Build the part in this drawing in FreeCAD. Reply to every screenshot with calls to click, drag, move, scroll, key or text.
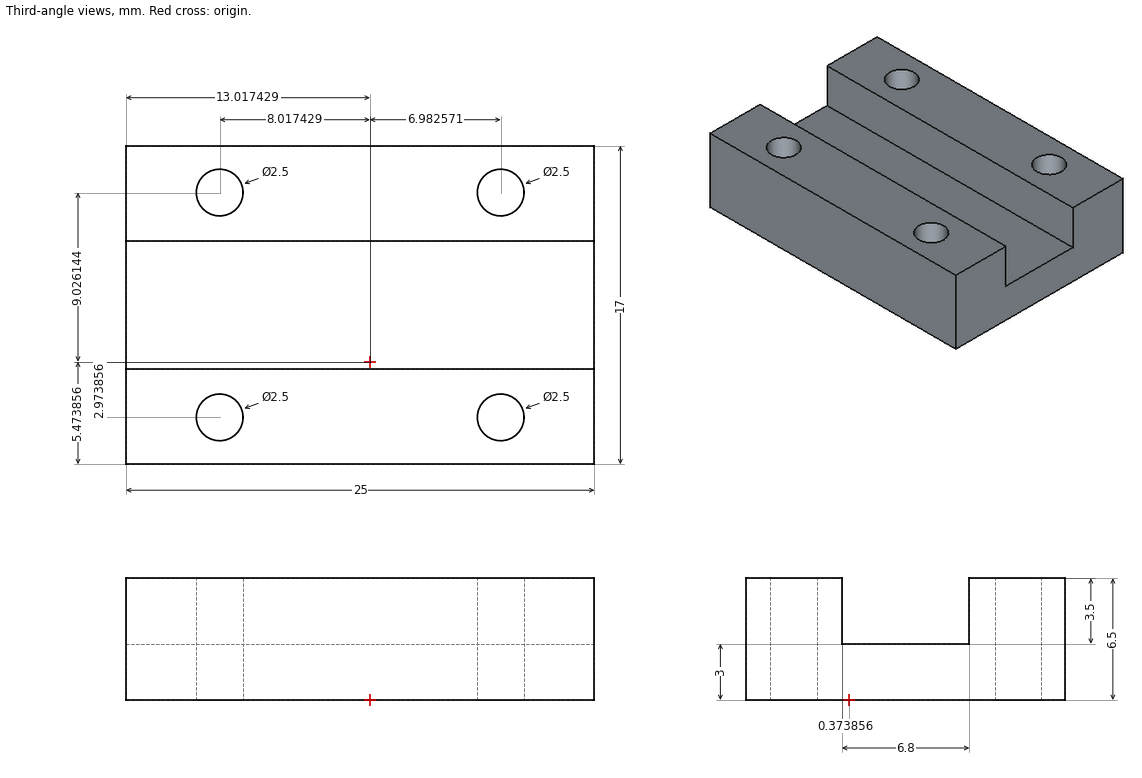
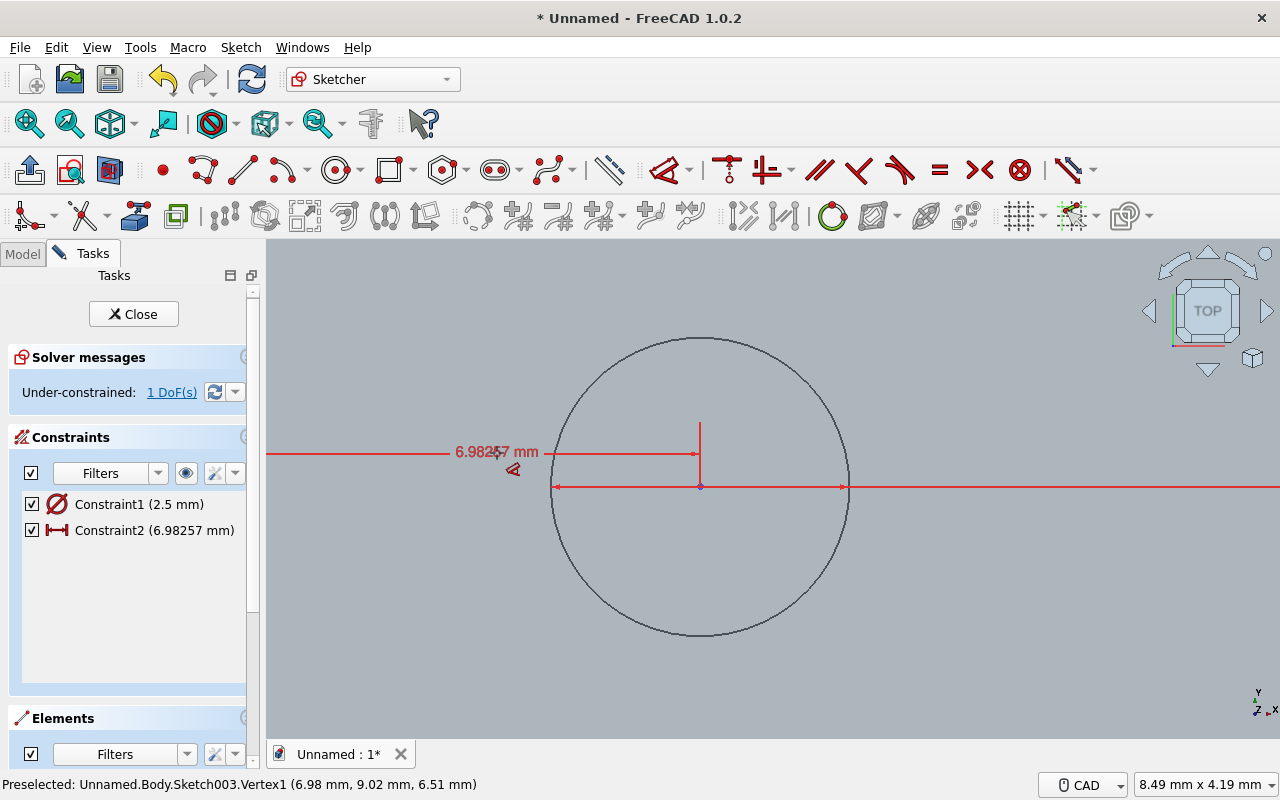
click(700, 487)
click(734, 599)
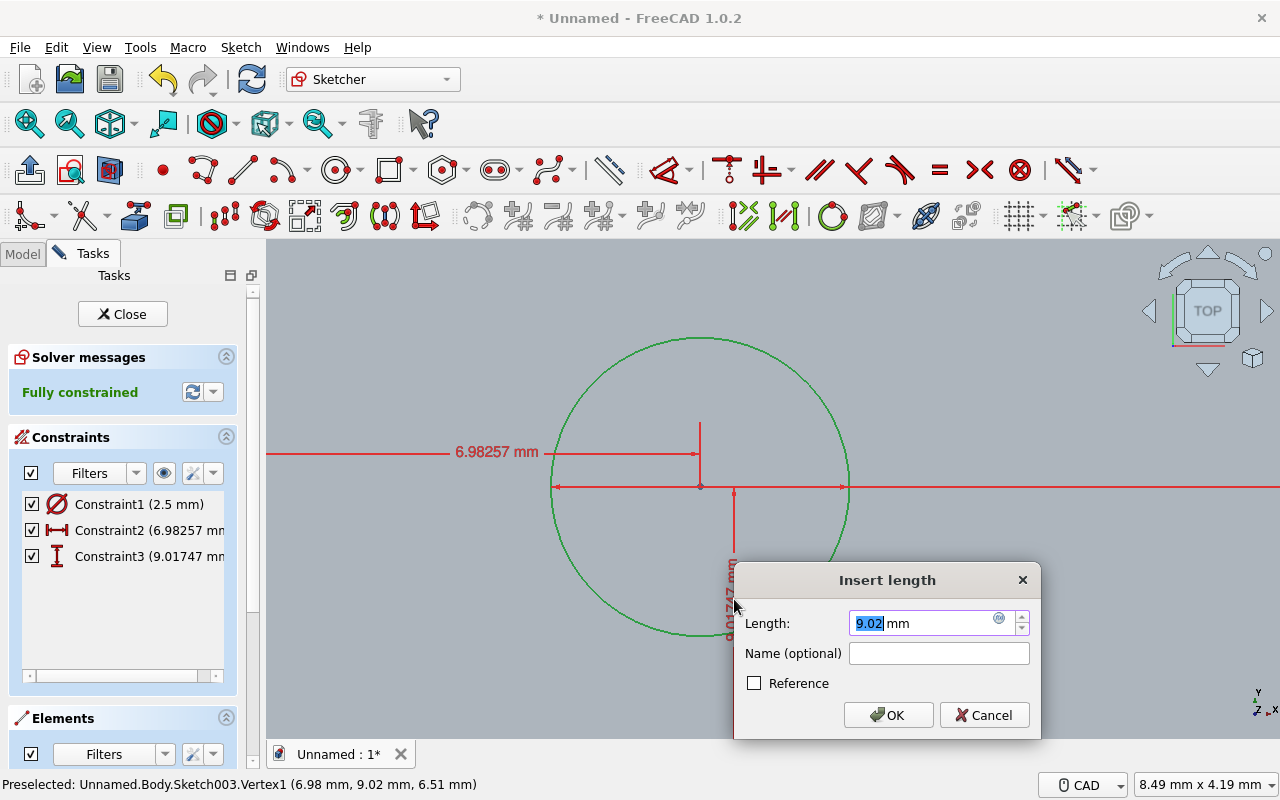
text(9.026144)
key(Return)
key(Escape)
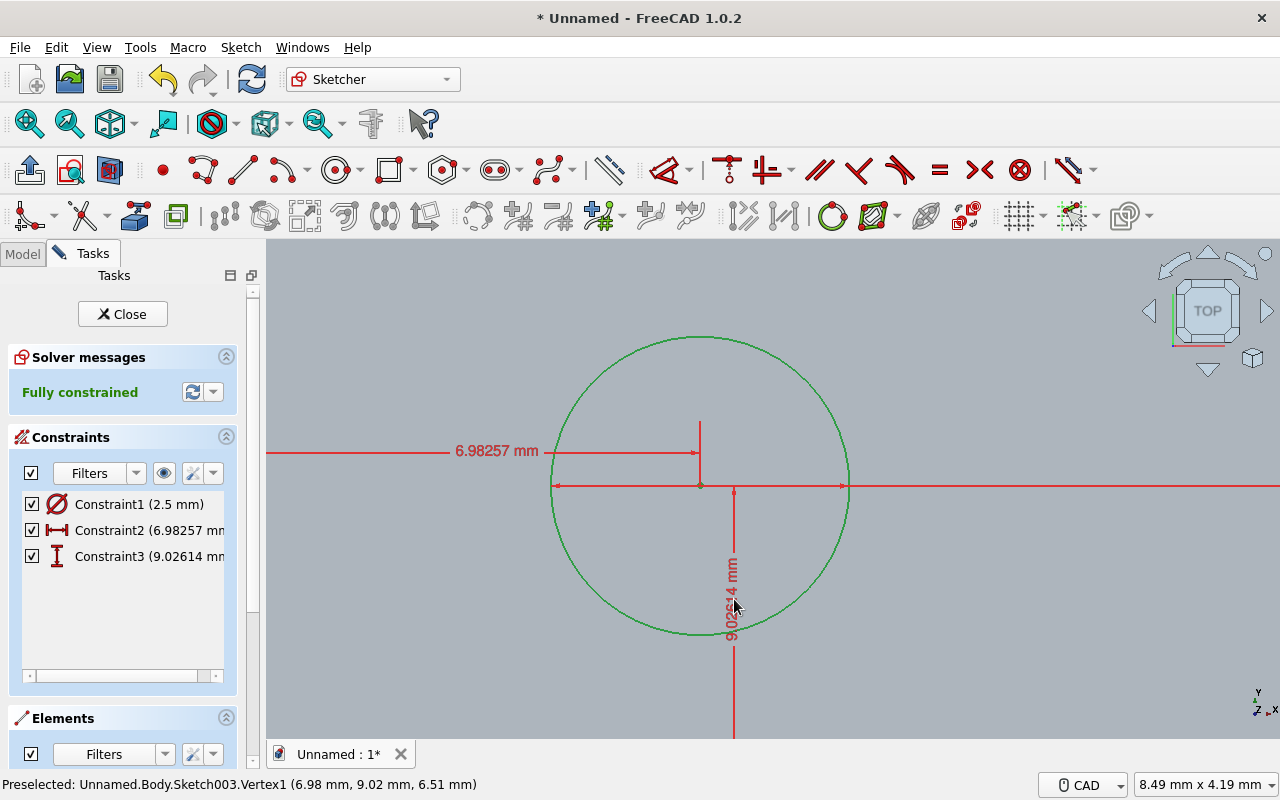
click(123, 314)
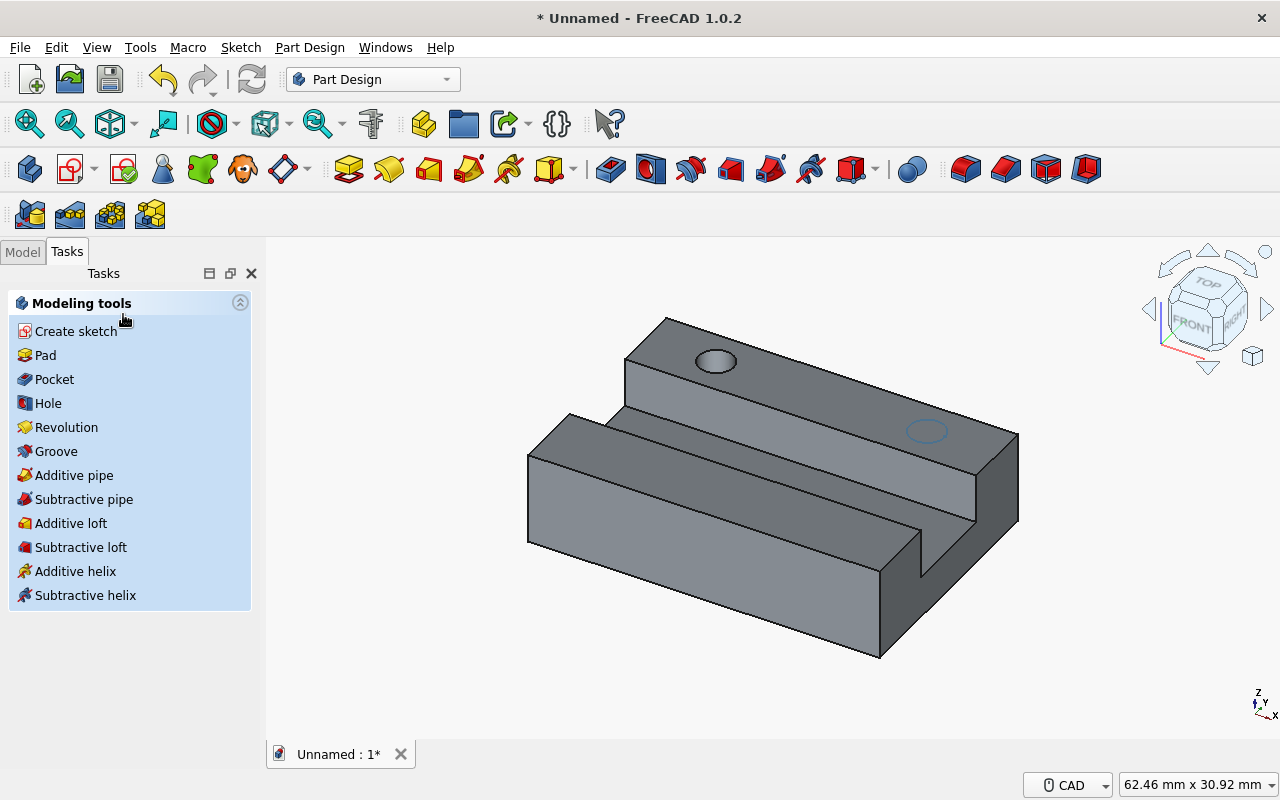
click(612, 170)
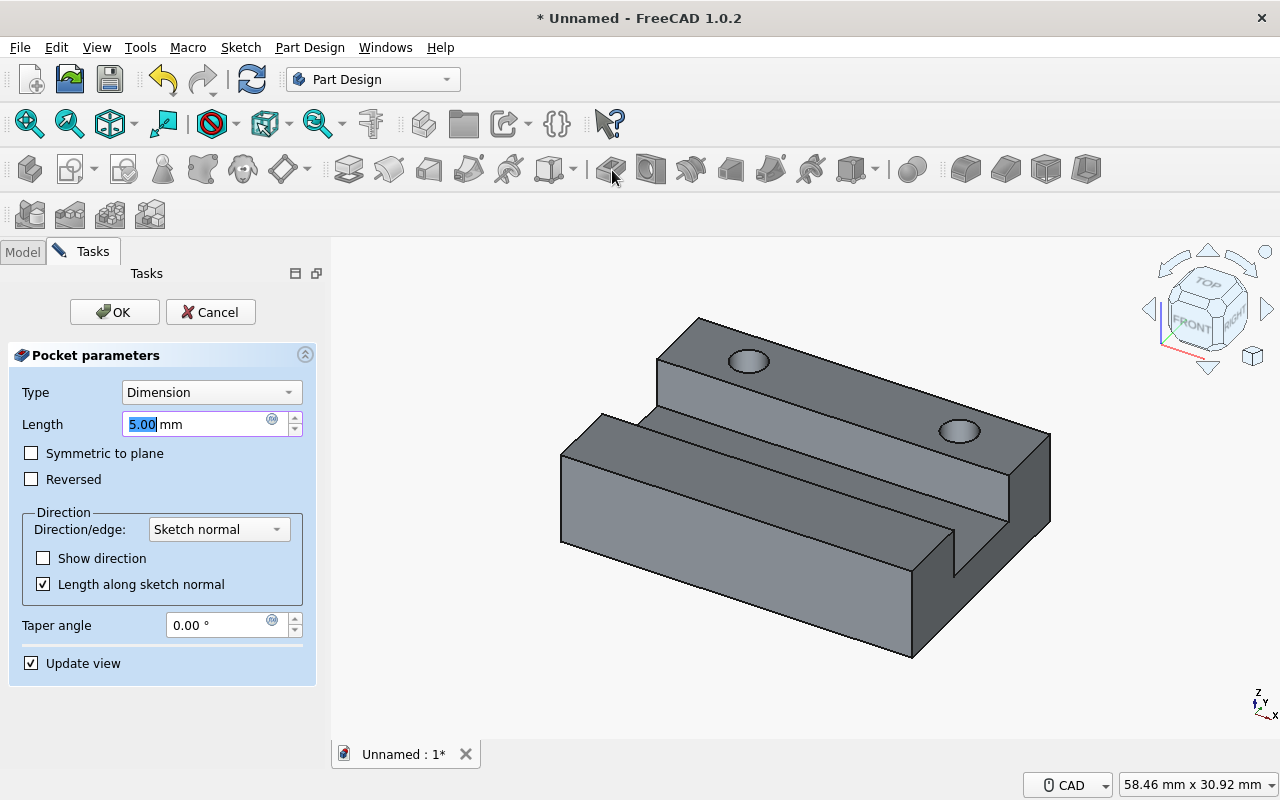
click(212, 392)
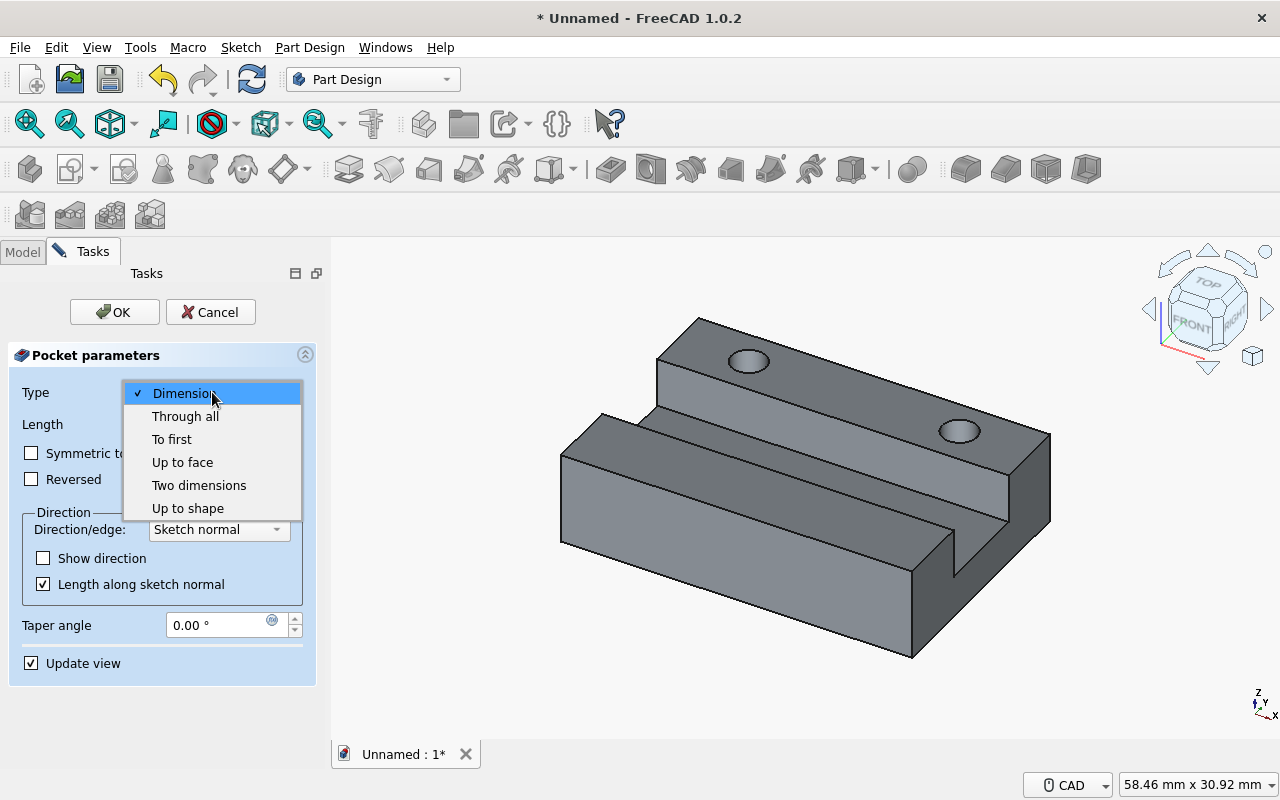
click(212, 440)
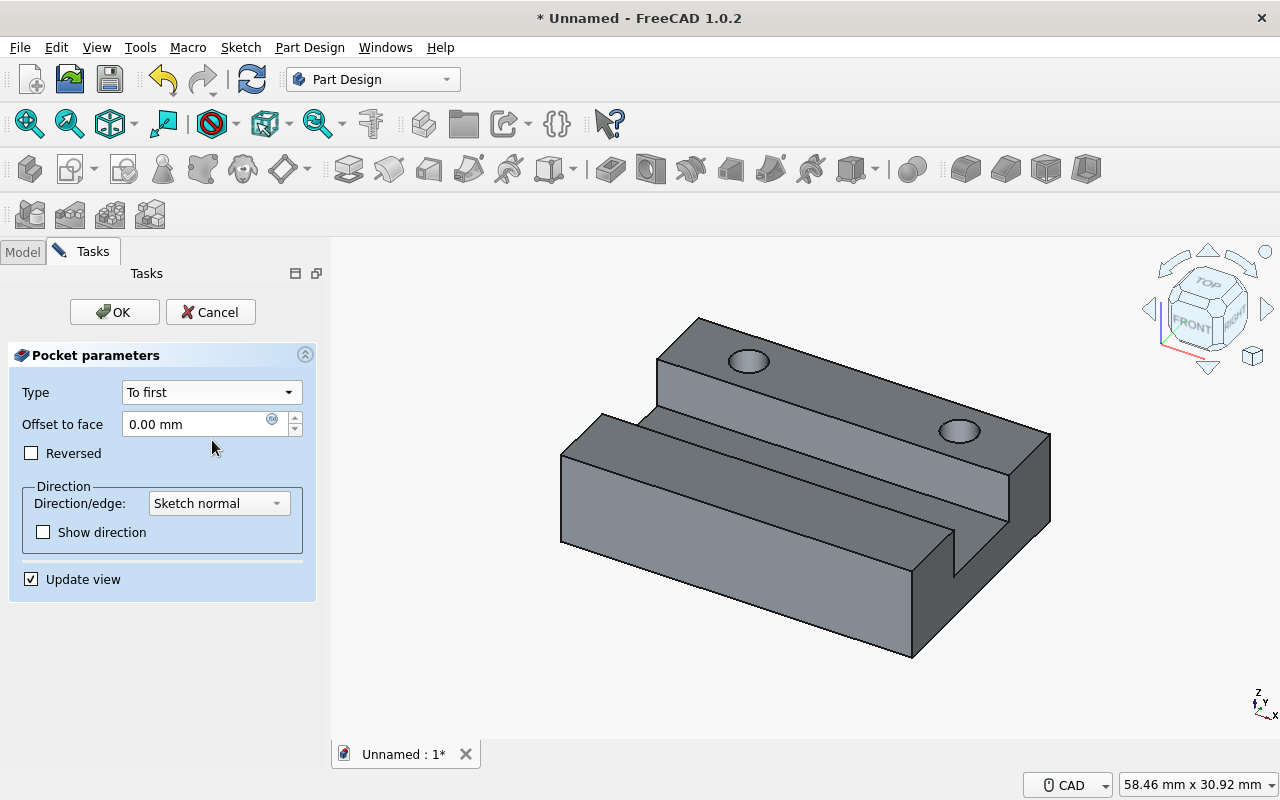
click(115, 312)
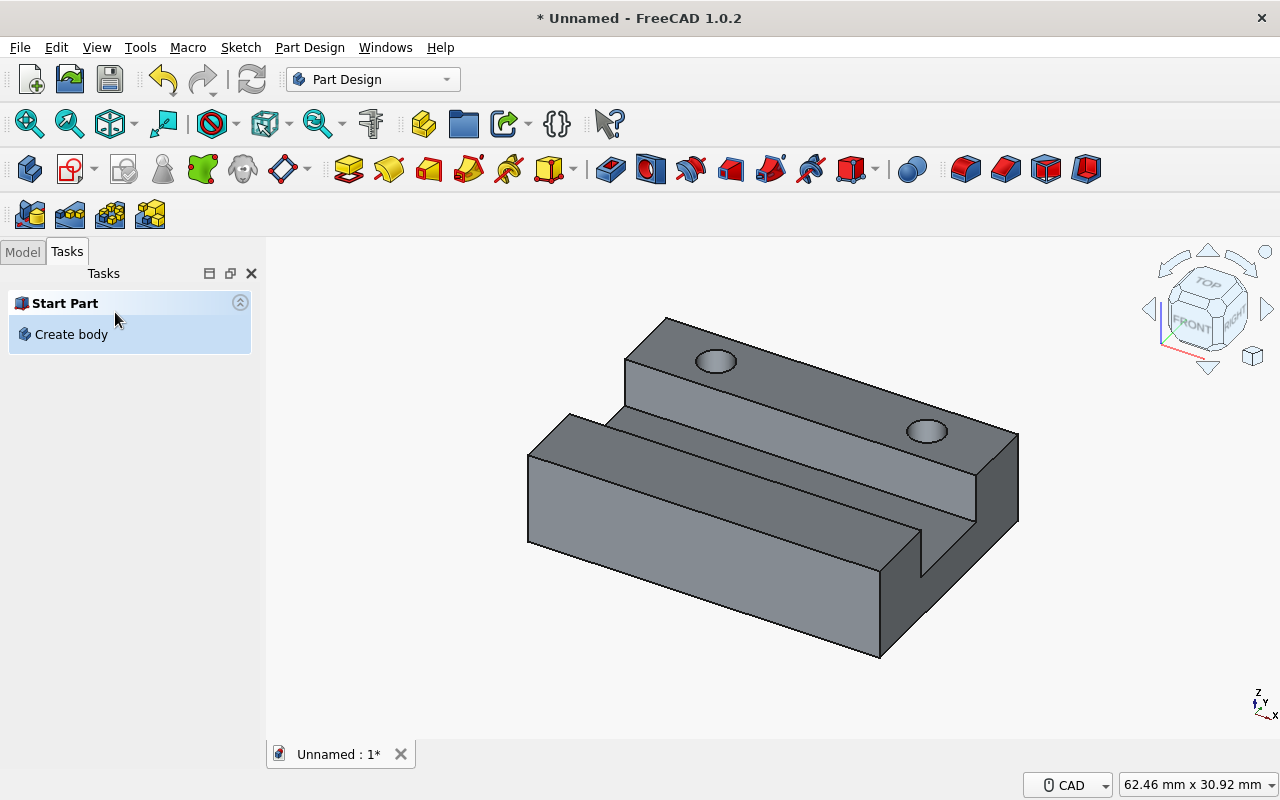
click(825, 525)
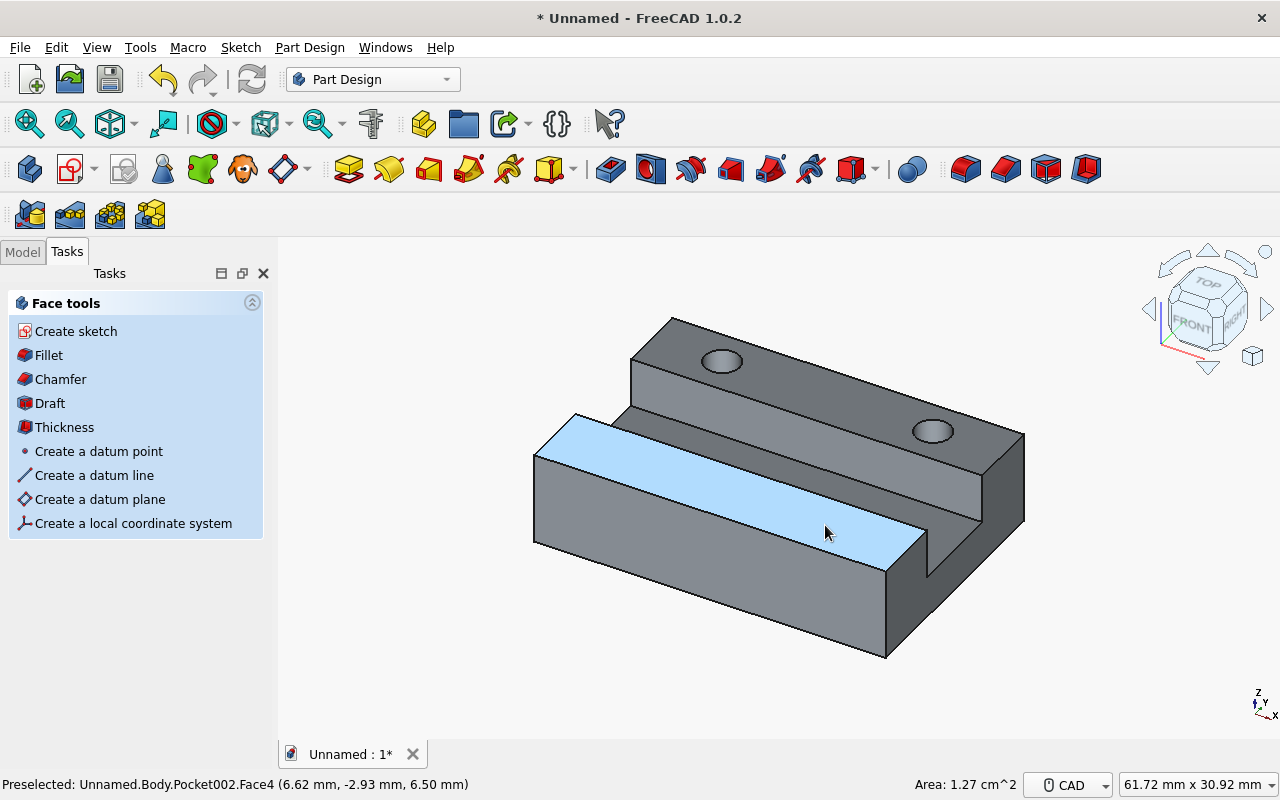
click(70, 170)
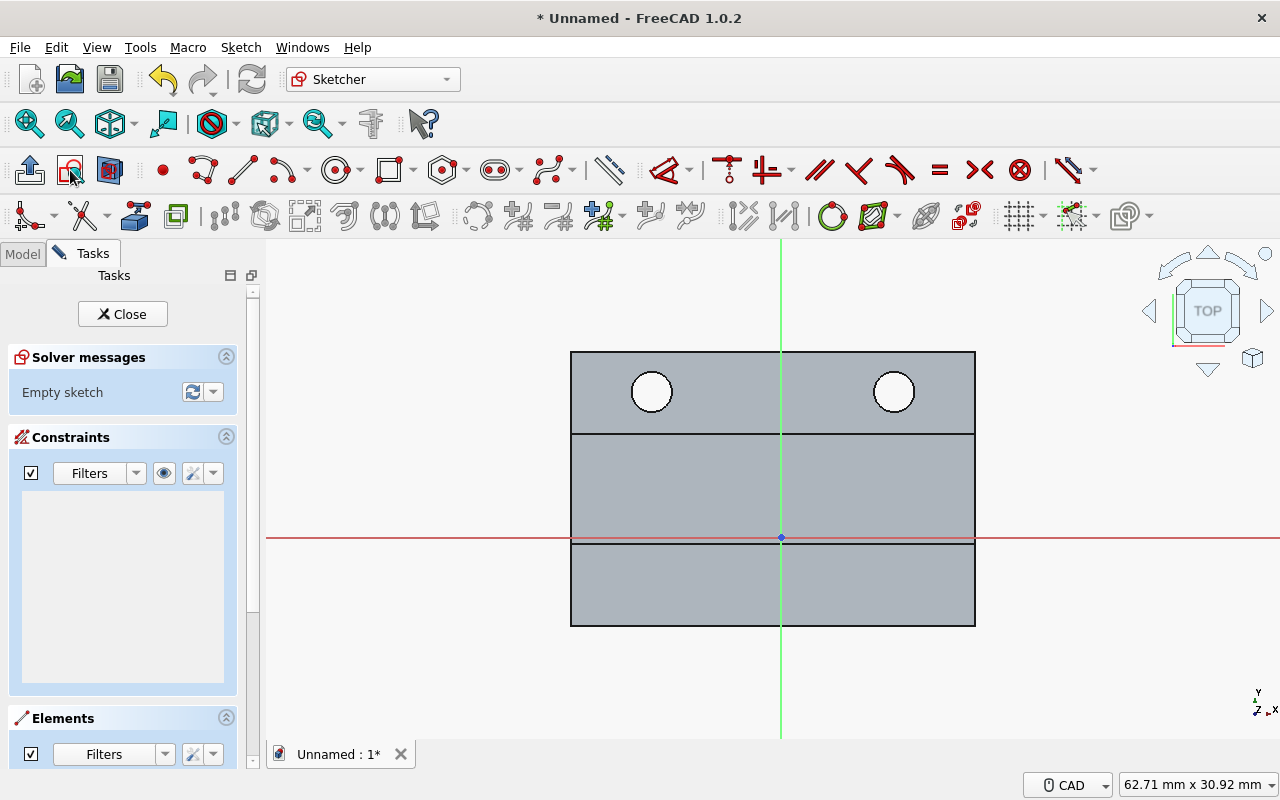
scroll(643, 601, up, 10)